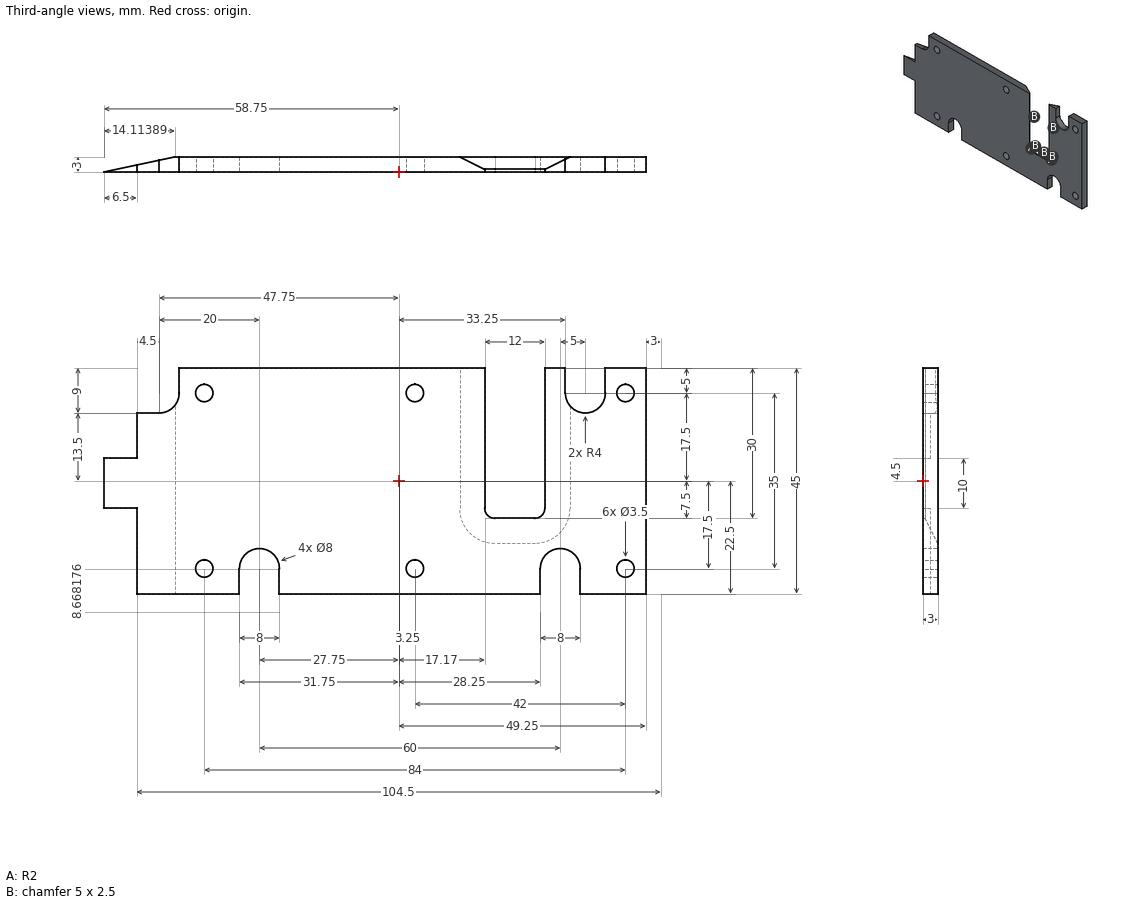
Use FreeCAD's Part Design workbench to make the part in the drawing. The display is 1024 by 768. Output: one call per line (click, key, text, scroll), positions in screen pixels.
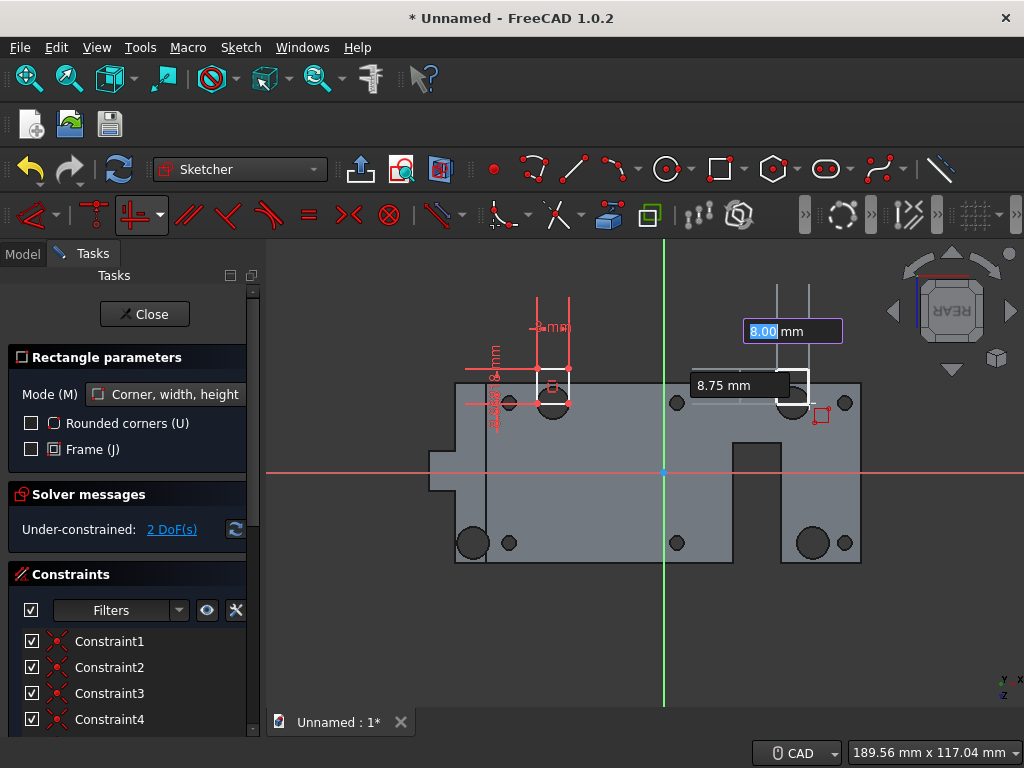
text(8)
key(Tab)
text(8.668176)
key(Return)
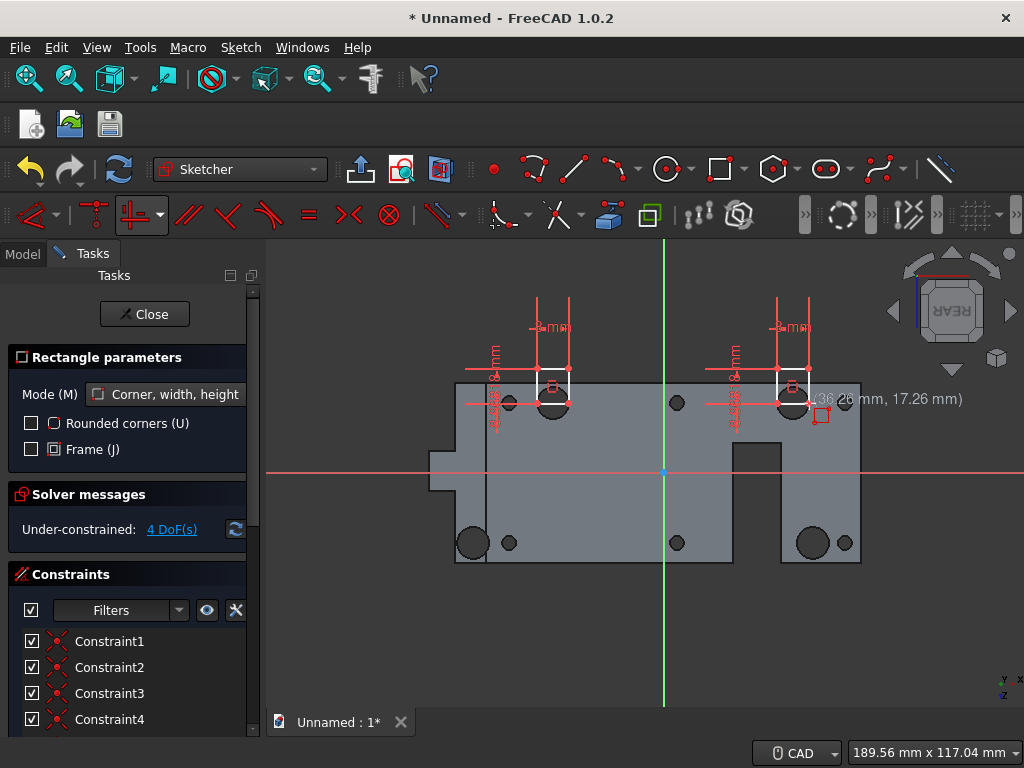
key(g)
key(m)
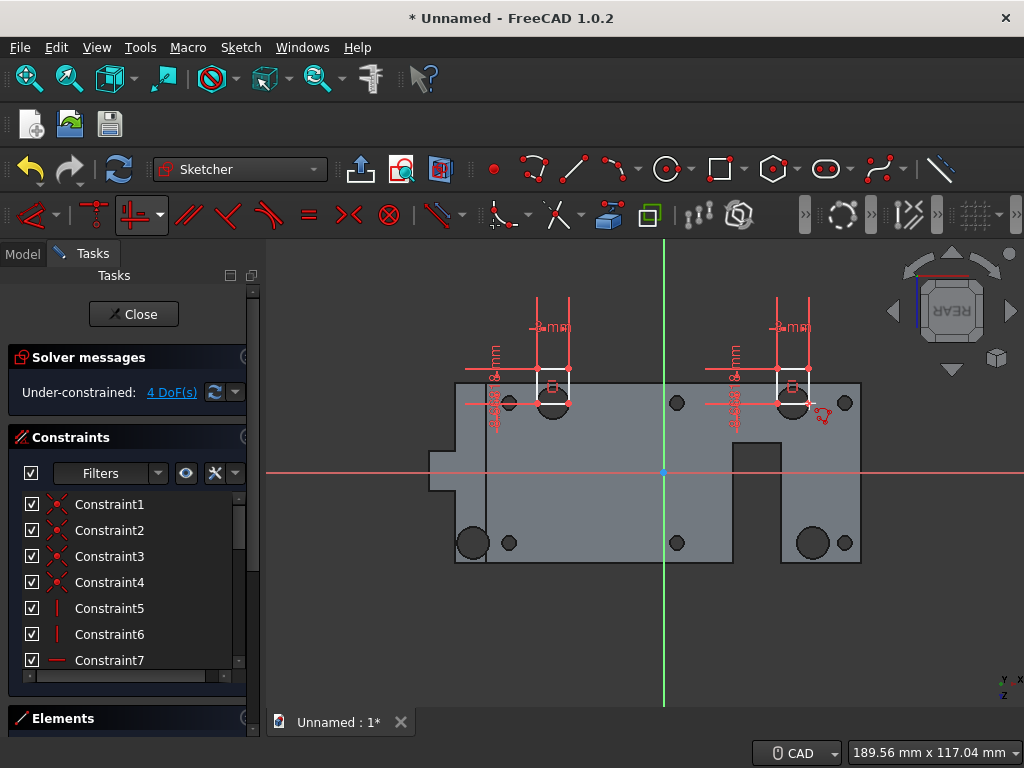
click(797, 543)
click(797, 563)
click(829, 563)
click(829, 543)
right_click(829, 543)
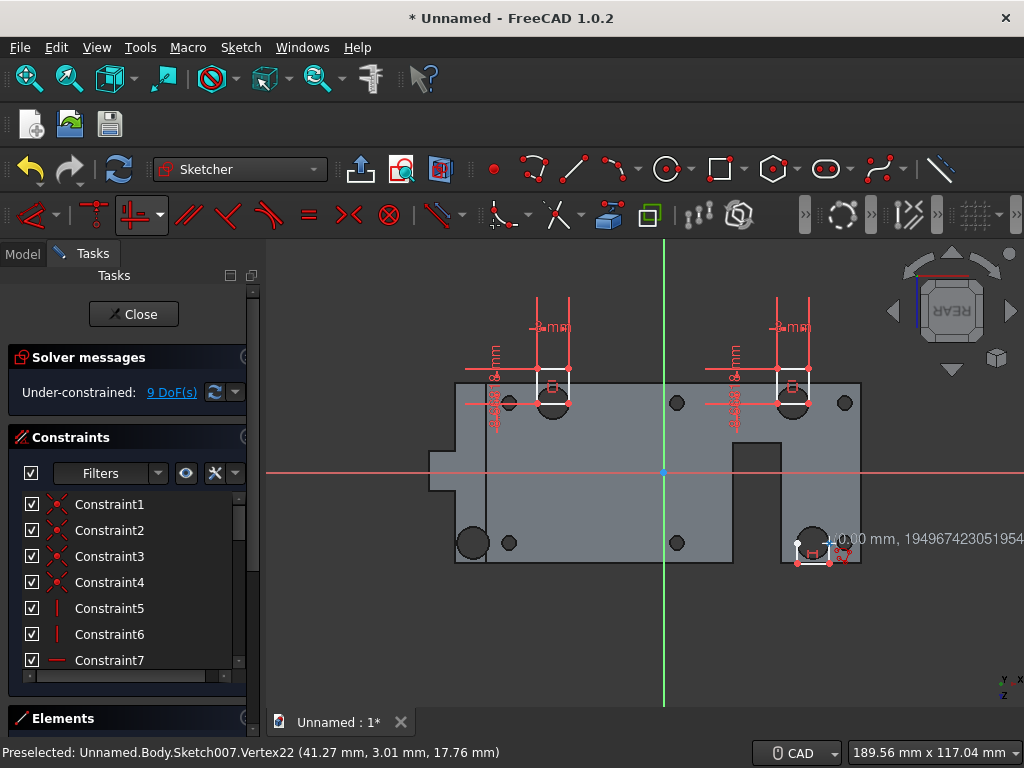
key(g)
key(3)
key(a)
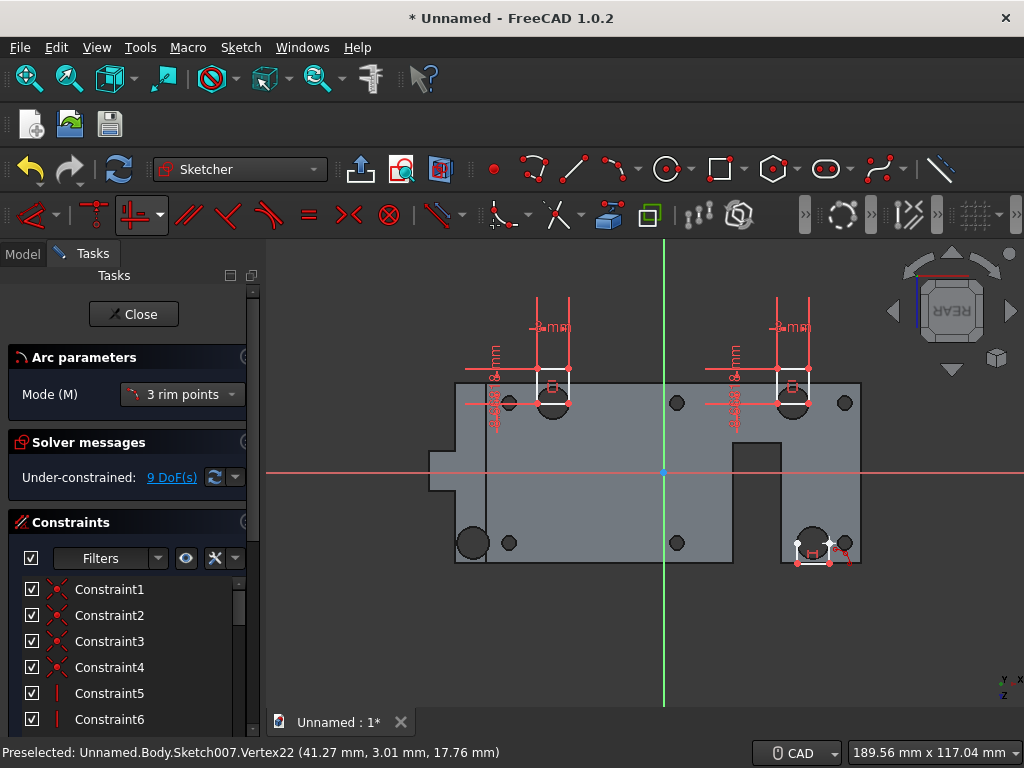
scroll(829, 543, up, 3)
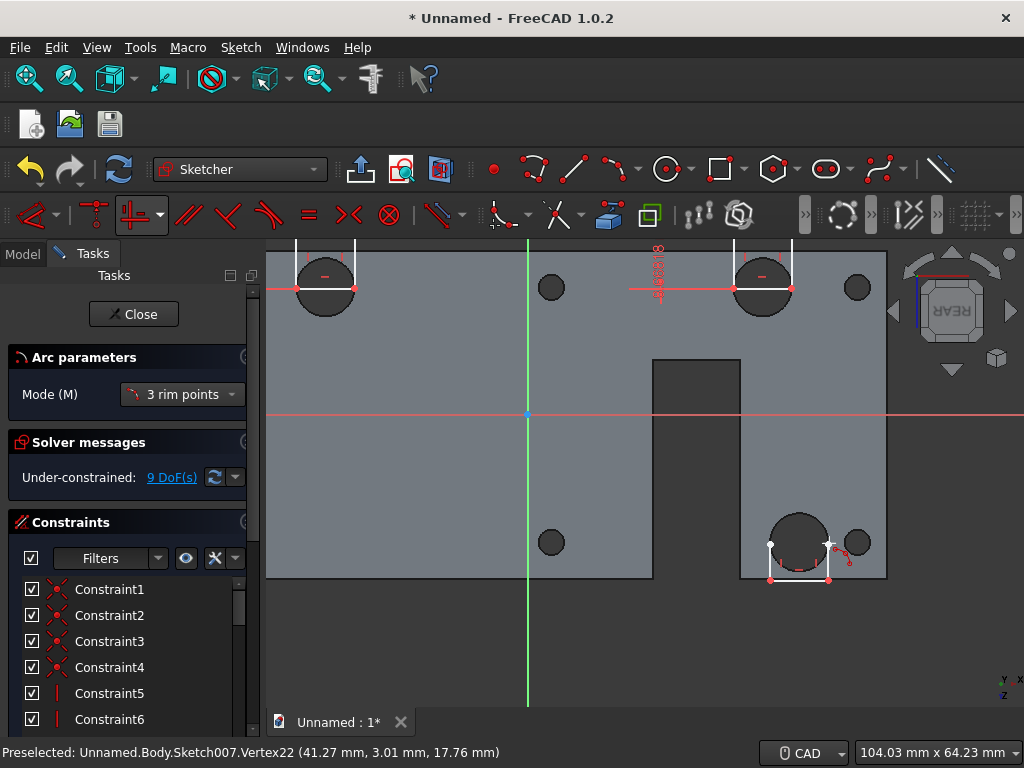
click(828, 544)
click(770, 544)
click(799, 513)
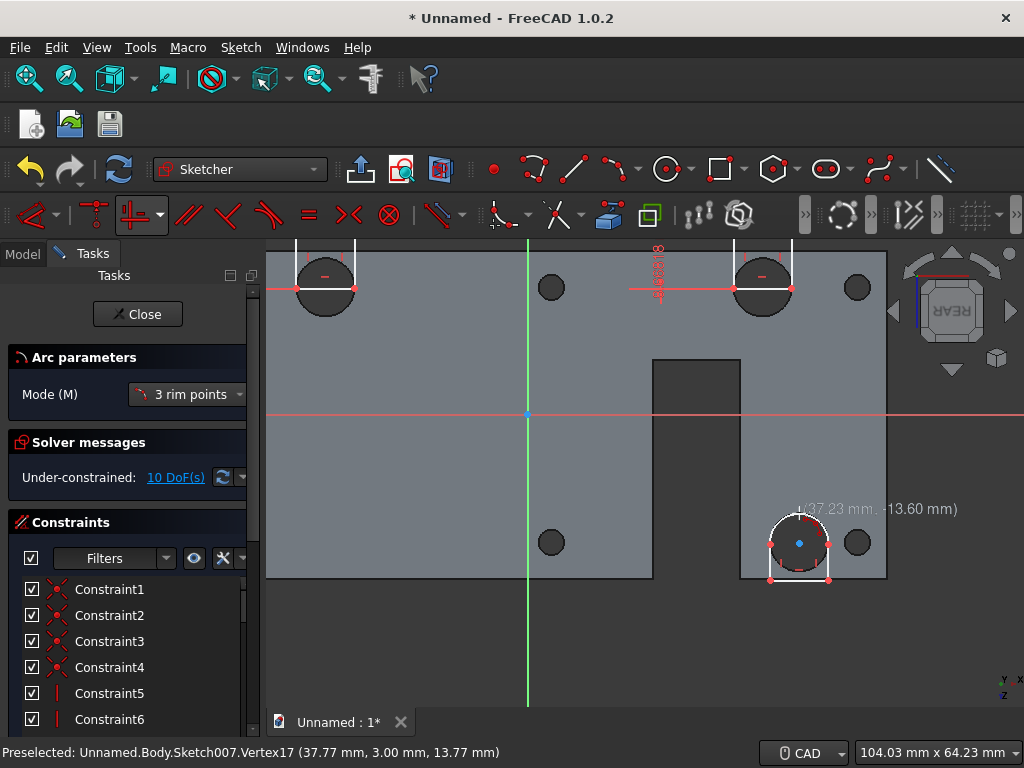
click(534, 170)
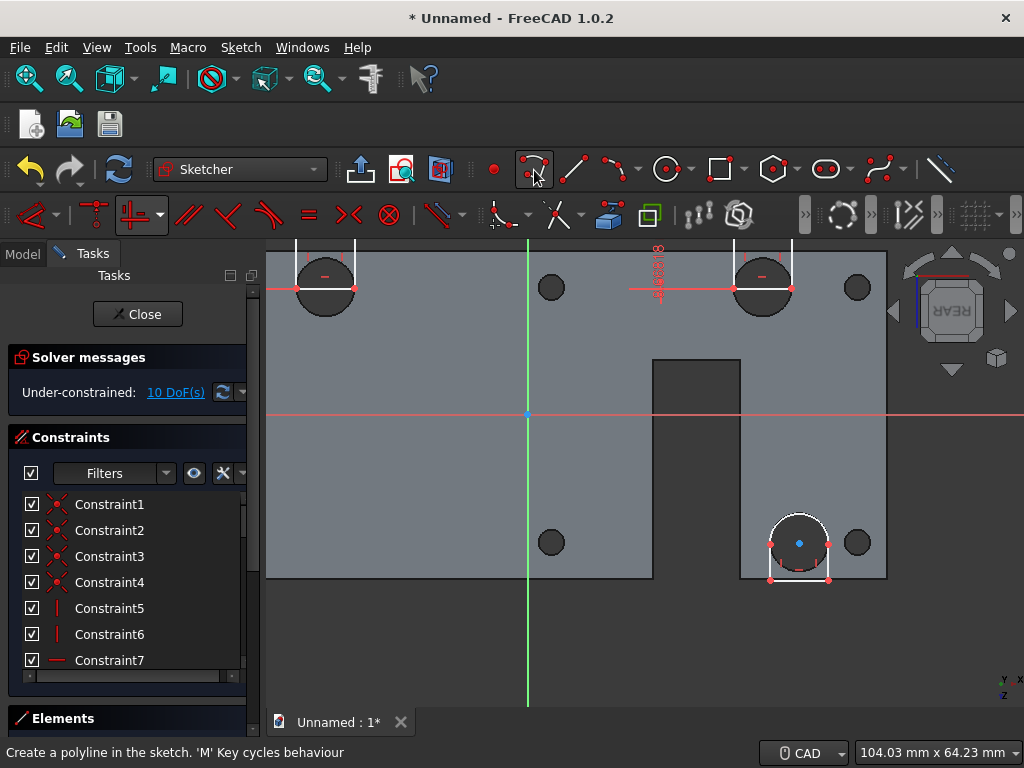
scroll(685, 560, down, 3)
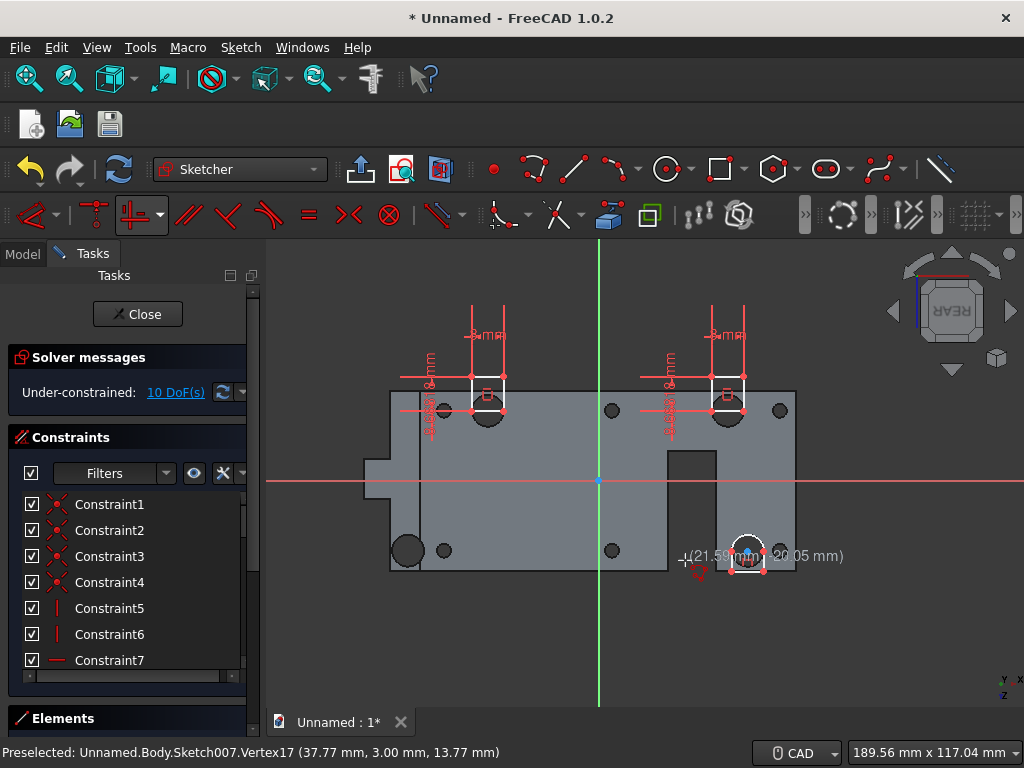
click(408, 535)
click(390, 535)
click(390, 571)
click(424, 571)
click(424, 551)
right_click(424, 551)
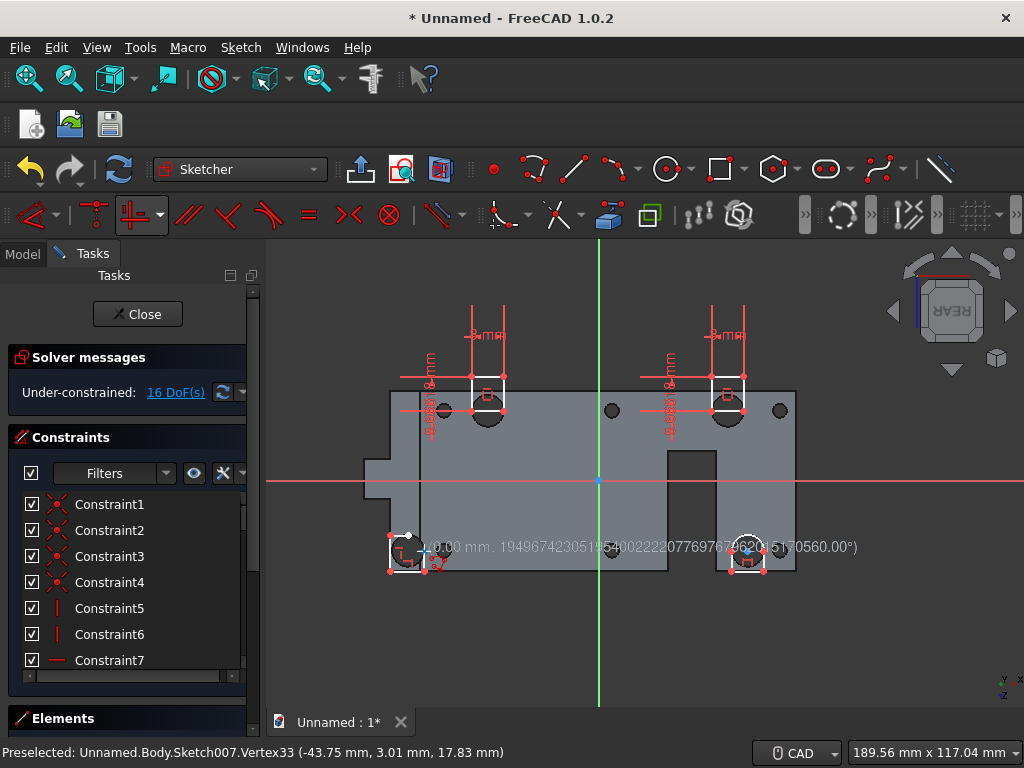
key(g)
key(3)
key(a)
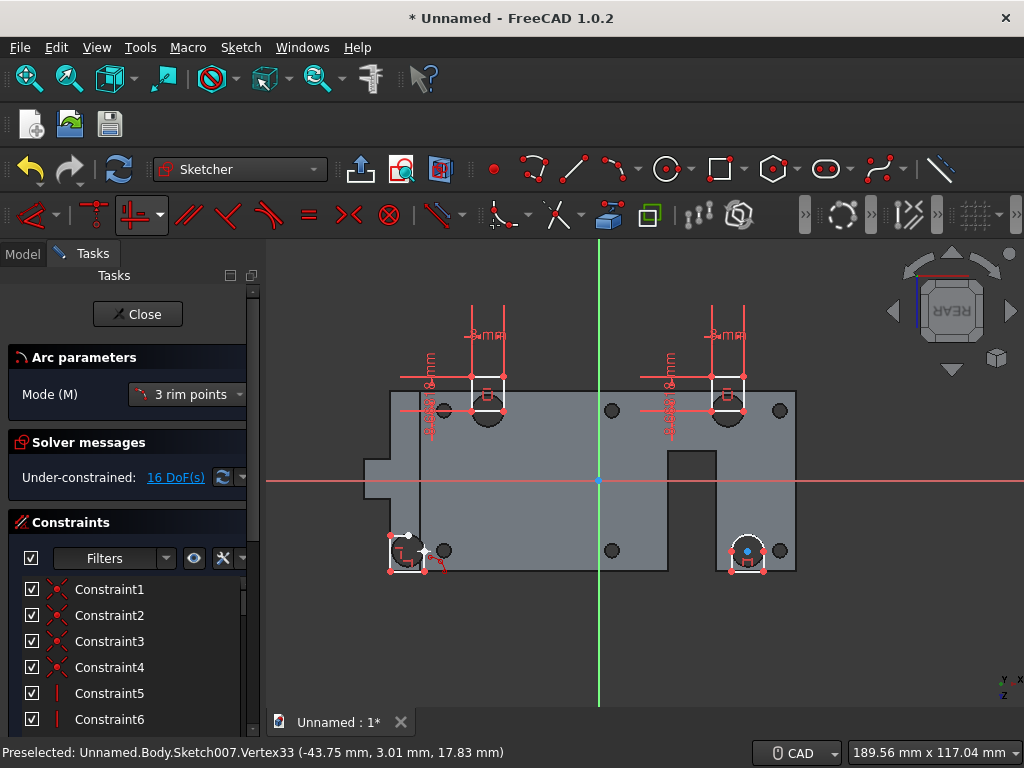
scroll(424, 551, up, 3)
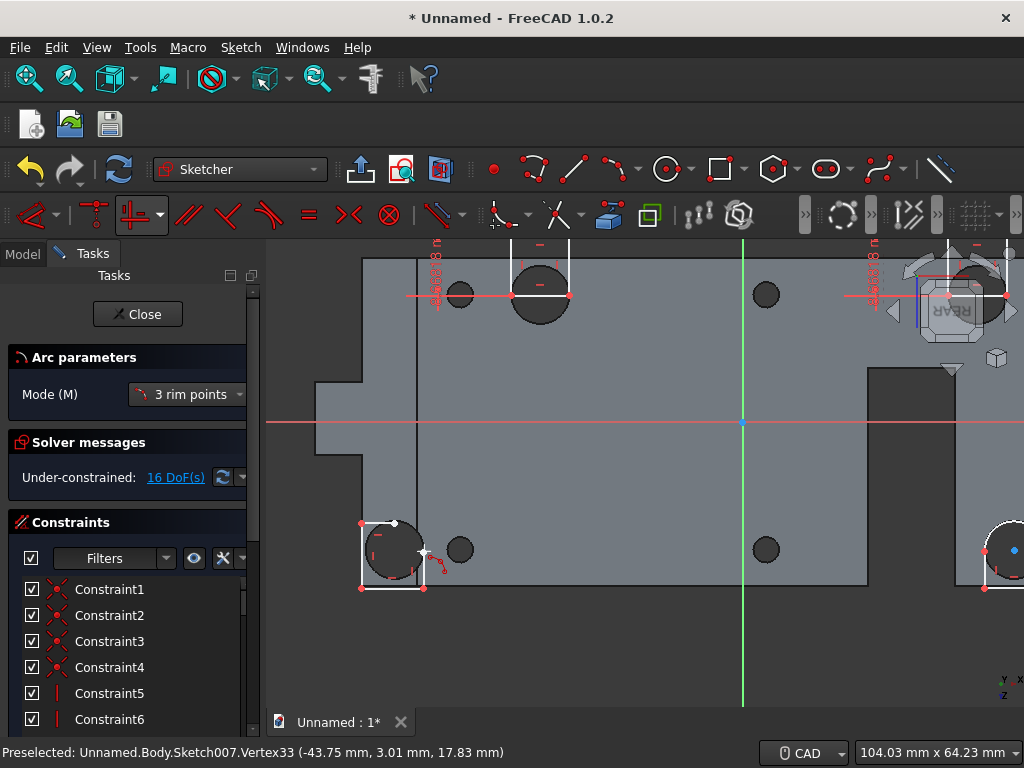
click(424, 552)
click(395, 523)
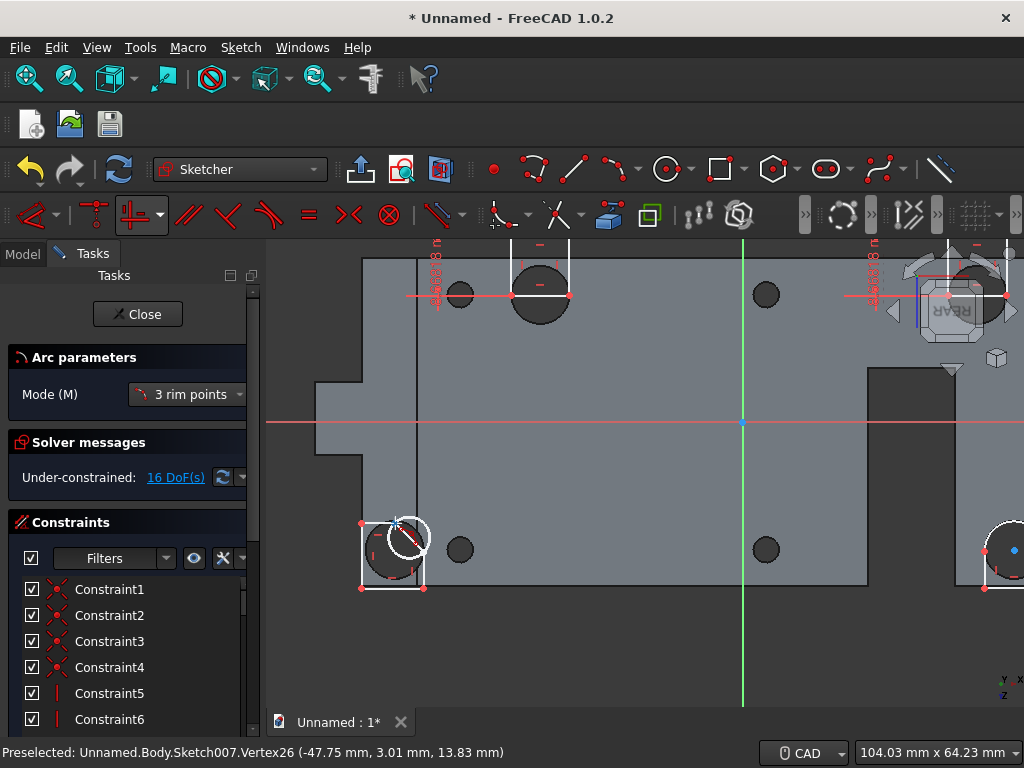
scroll(415, 529, up, 4)